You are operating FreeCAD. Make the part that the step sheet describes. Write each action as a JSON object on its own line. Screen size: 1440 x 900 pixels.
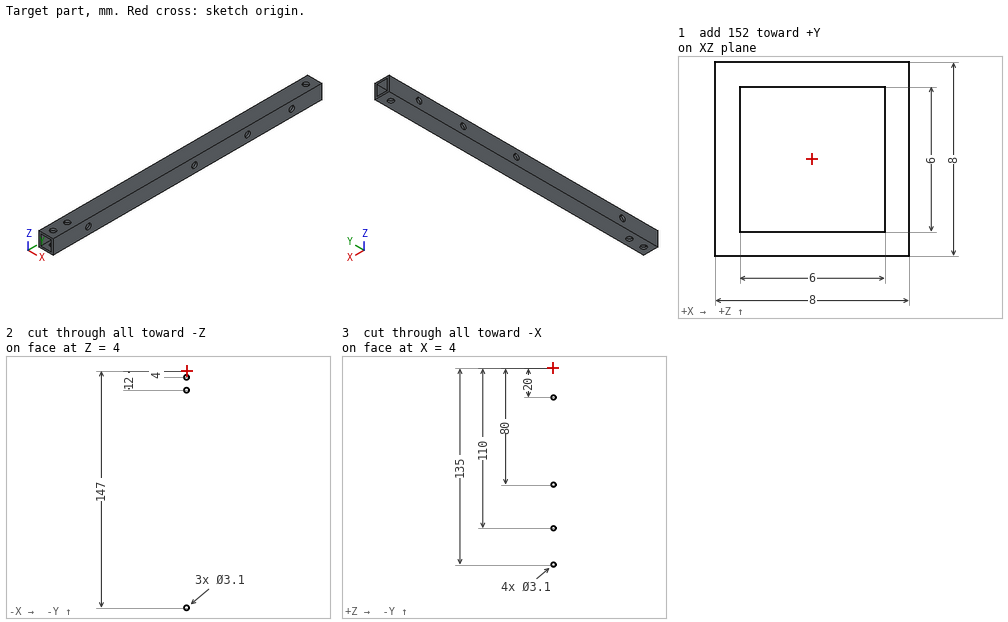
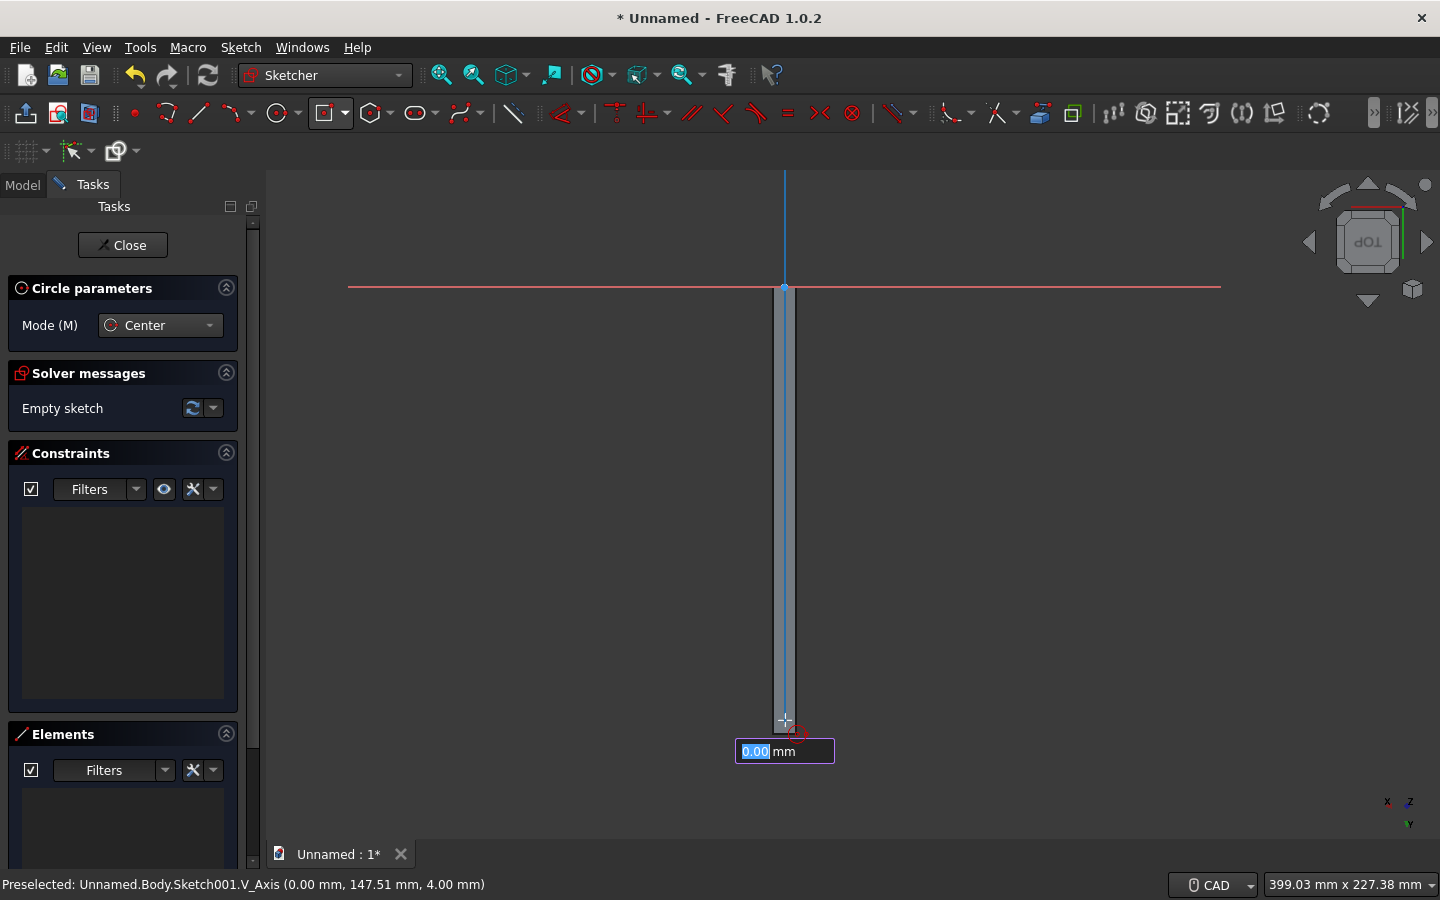
{"action": "scroll", "coordinate": [789, 718], "scroll_direction": "up", "scroll_amount": 7}
{"action": "mouse_move", "coordinate": [787, 715]}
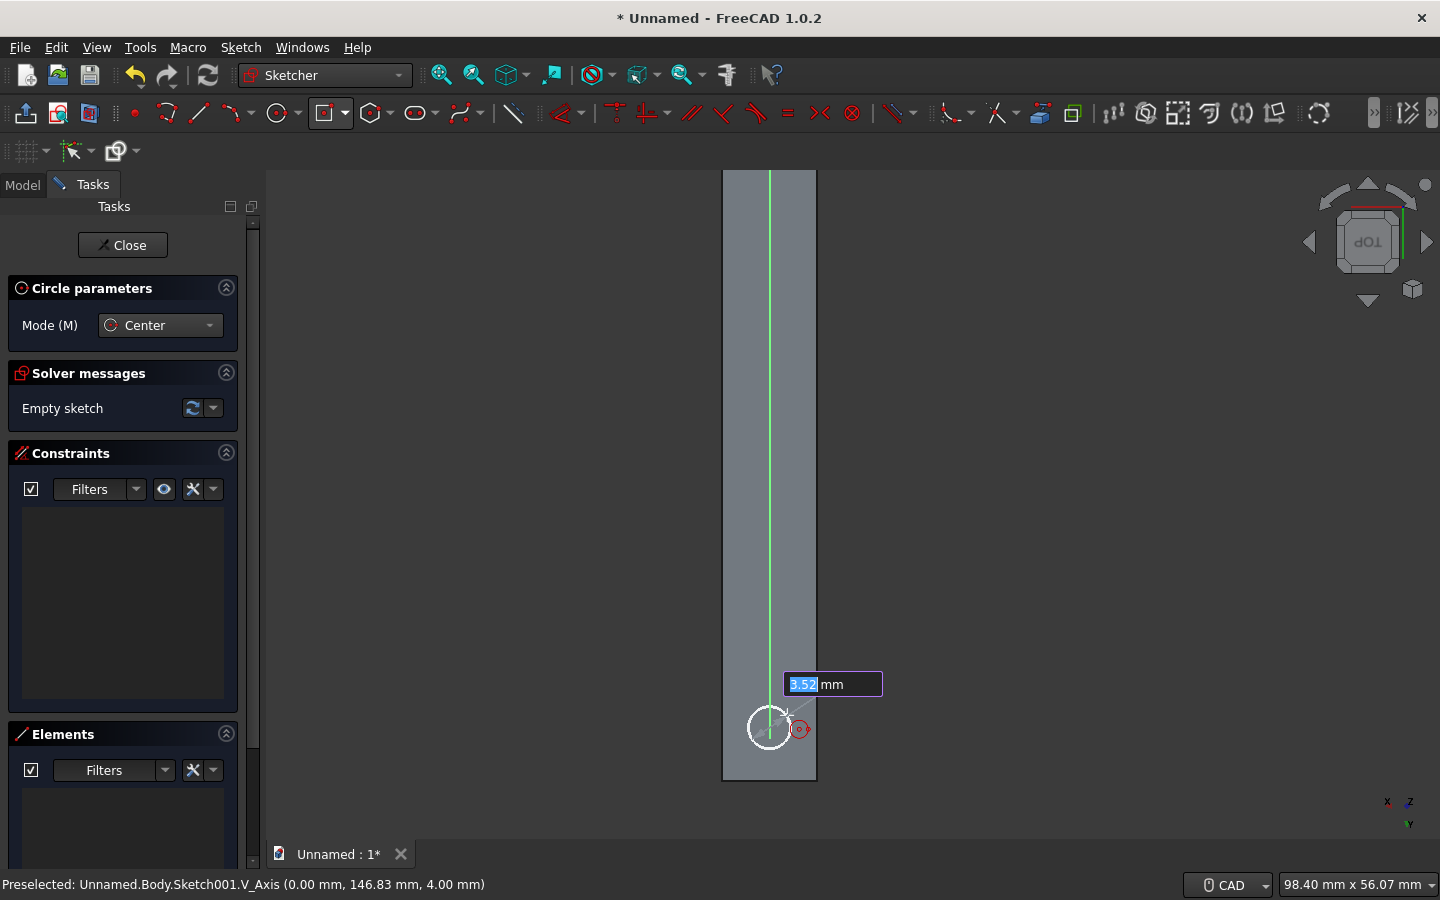
{"action": "type", "text": "3.1"}
{"action": "key", "text": "Return"}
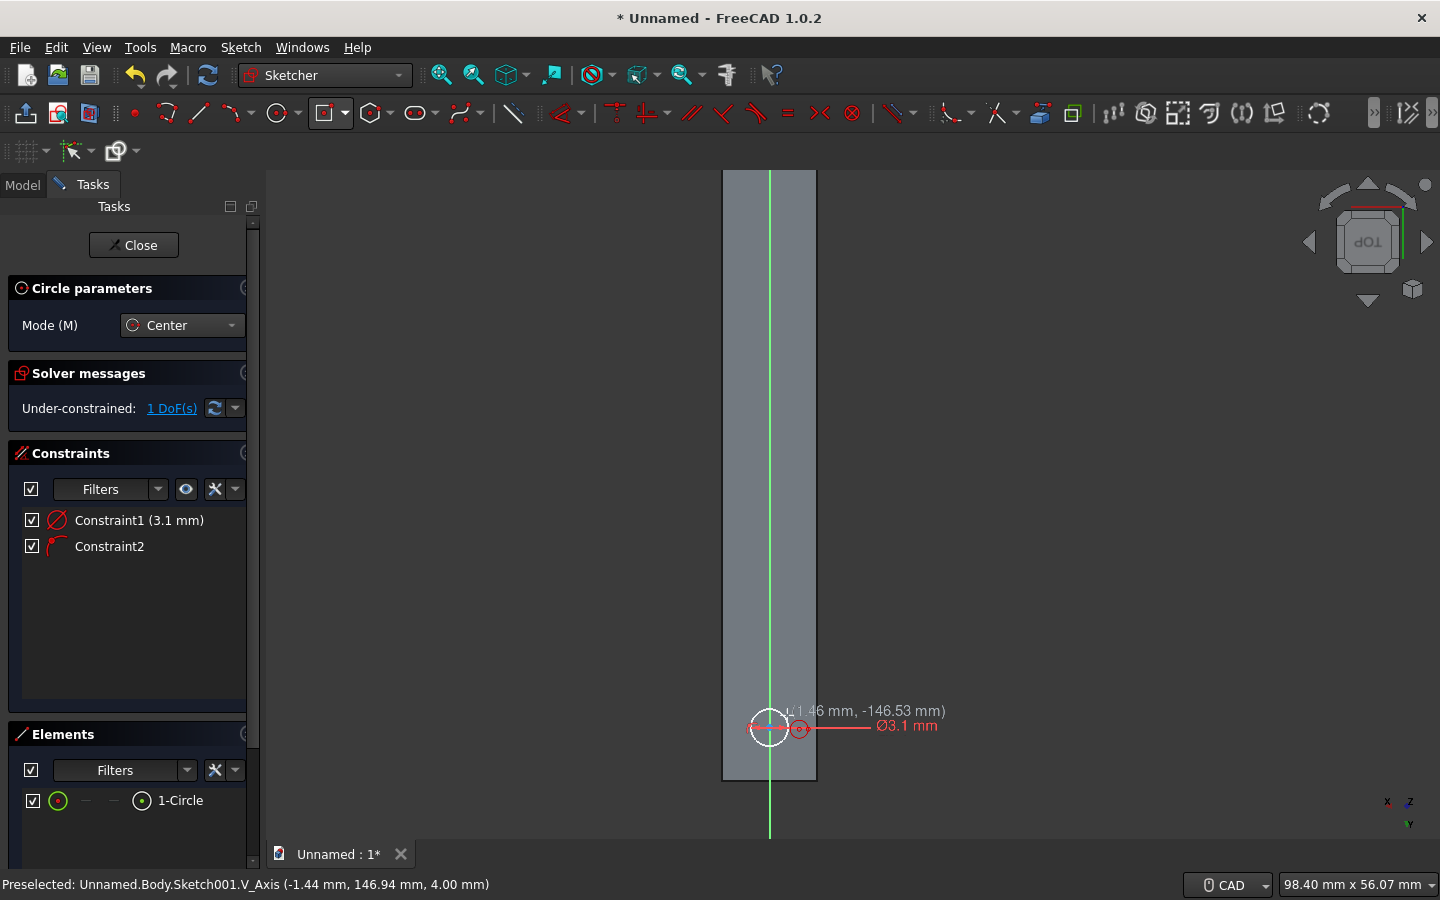
{"action": "scroll", "coordinate": [789, 717], "scroll_direction": "down", "scroll_amount": 7}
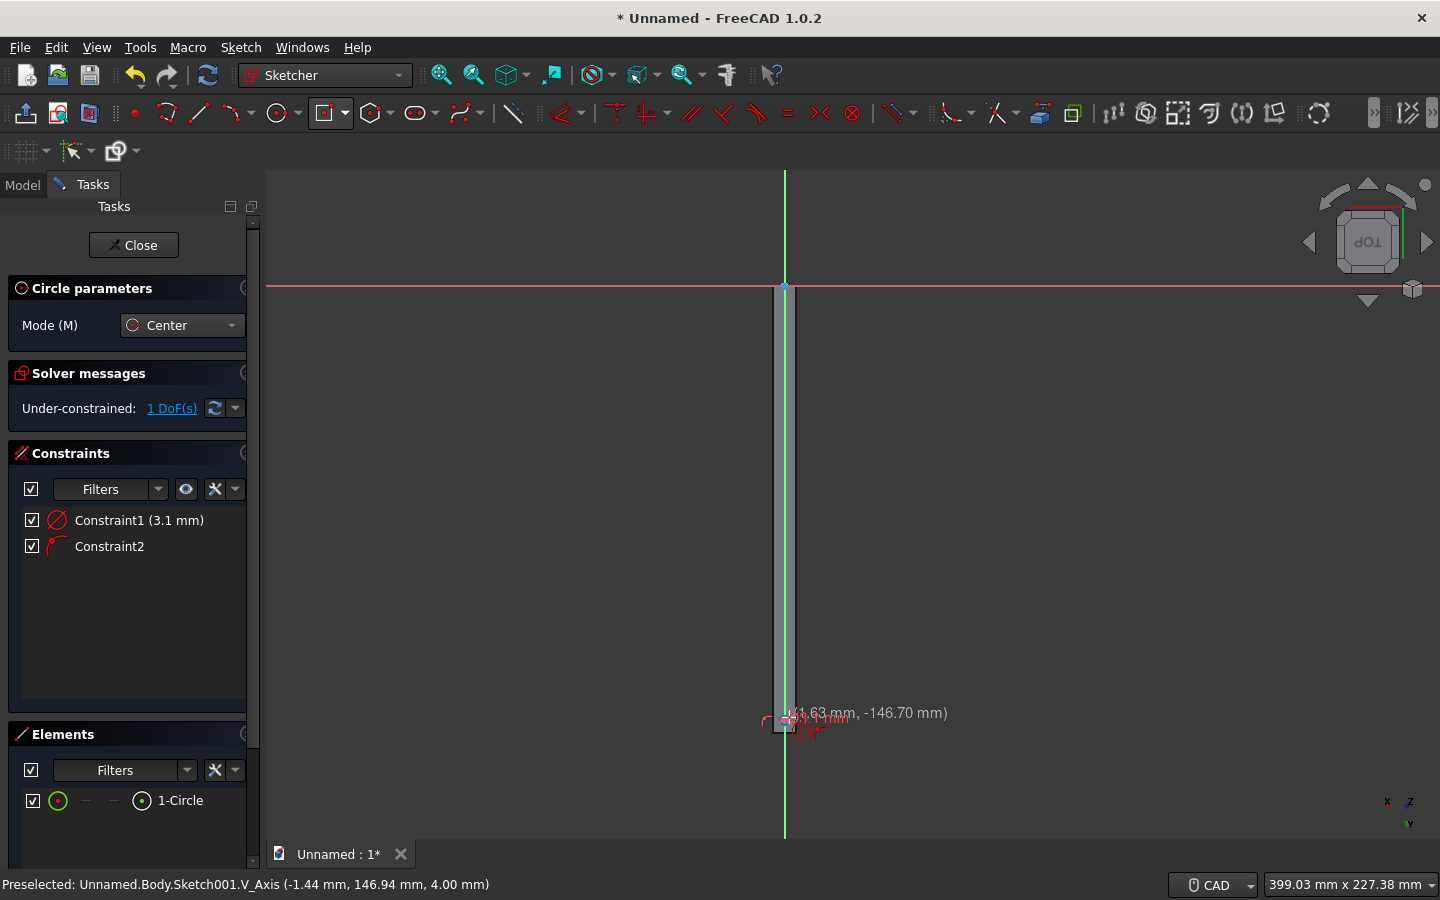
{"action": "scroll", "coordinate": [785, 298], "scroll_direction": "up", "scroll_amount": 9}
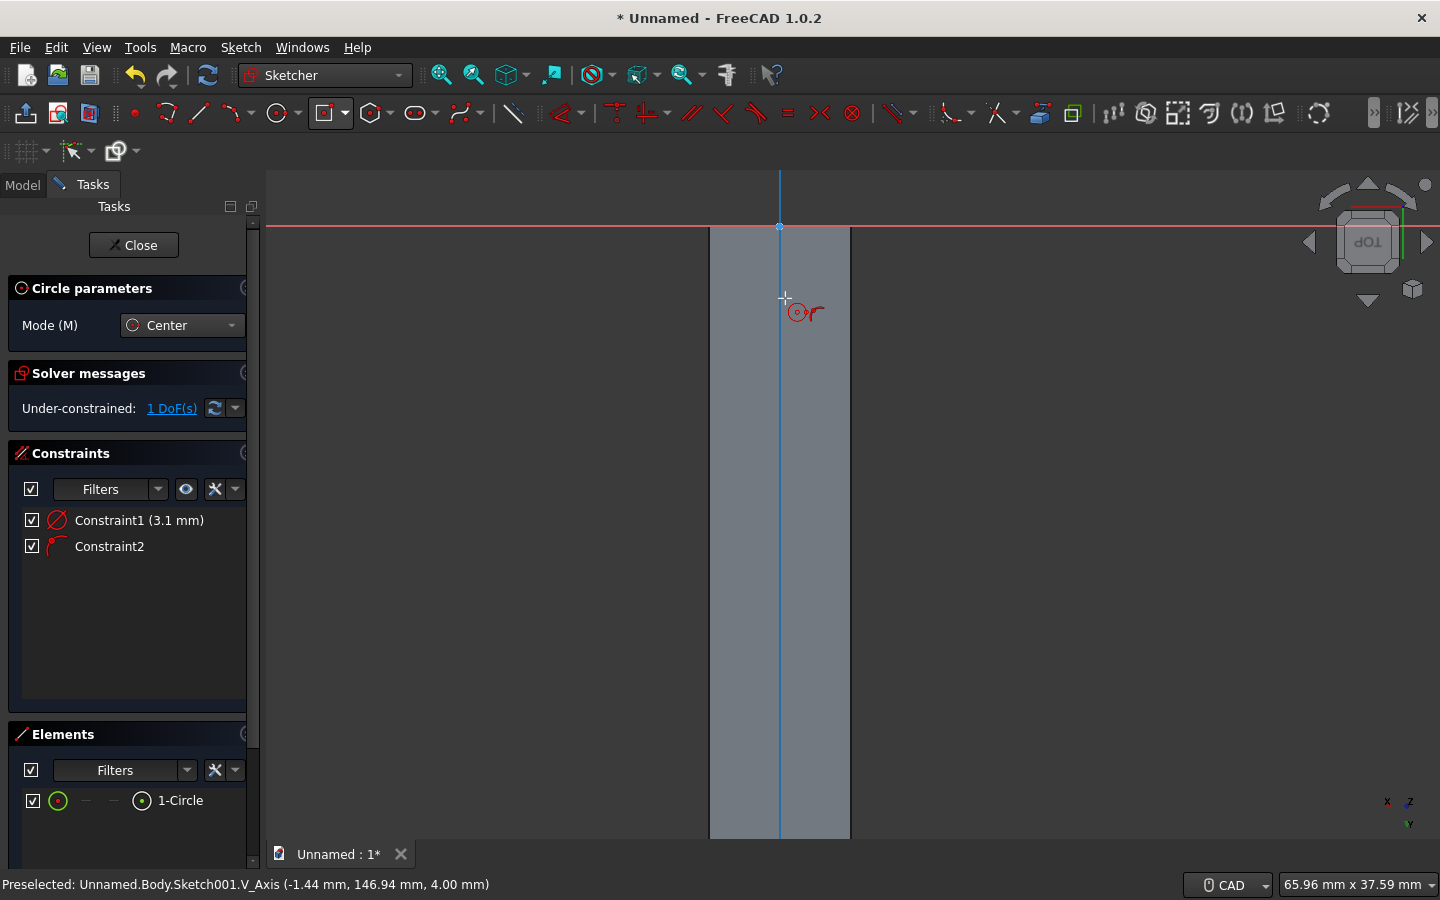
{"action": "scroll", "coordinate": [785, 298], "scroll_direction": "down", "scroll_amount": 9}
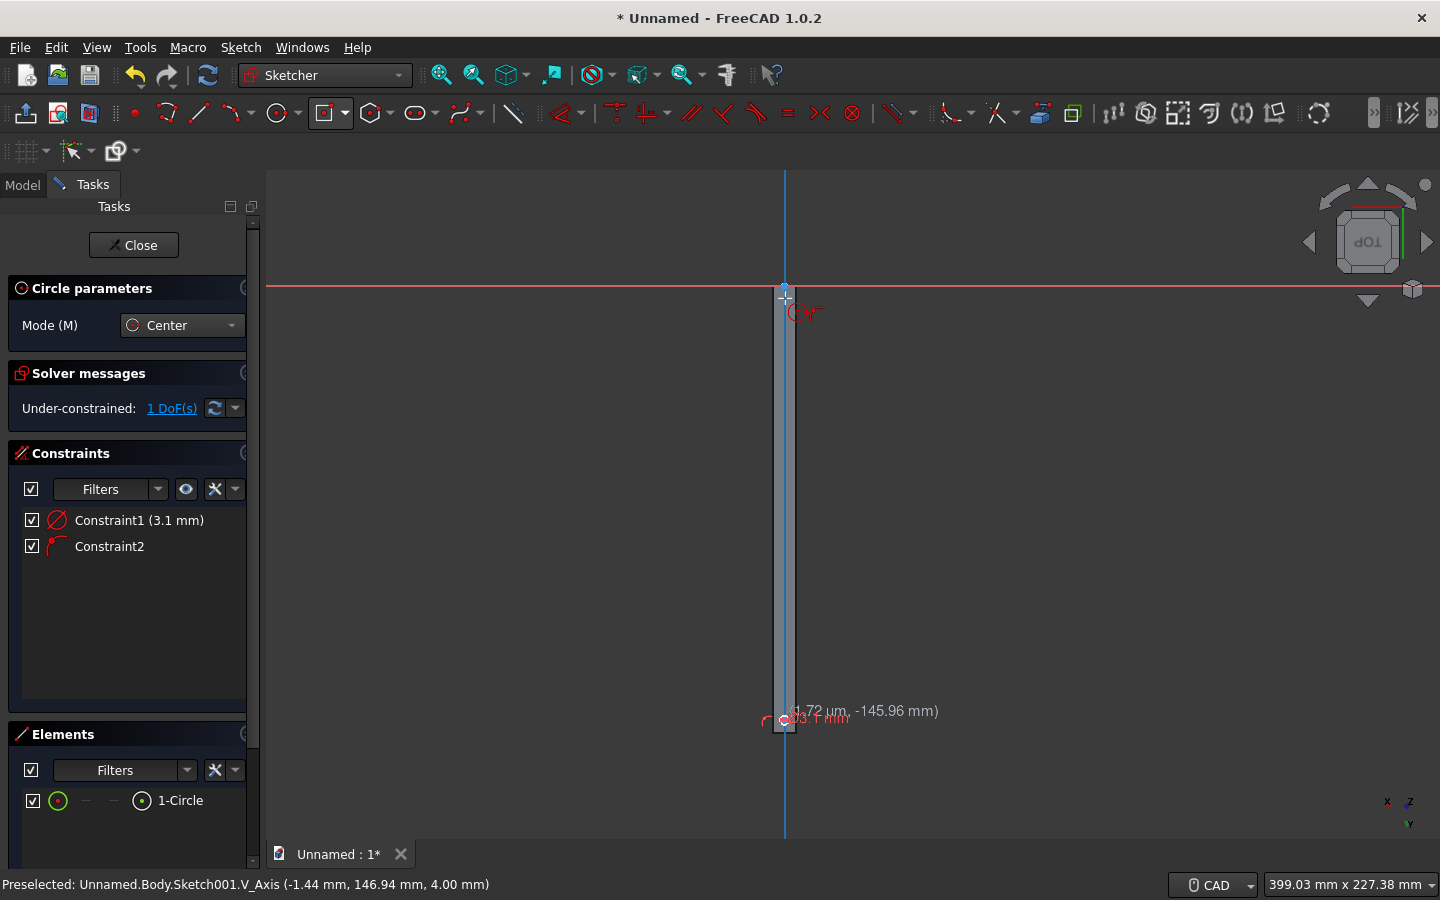
{"action": "scroll", "coordinate": [785, 298], "scroll_direction": "up", "scroll_amount": 2}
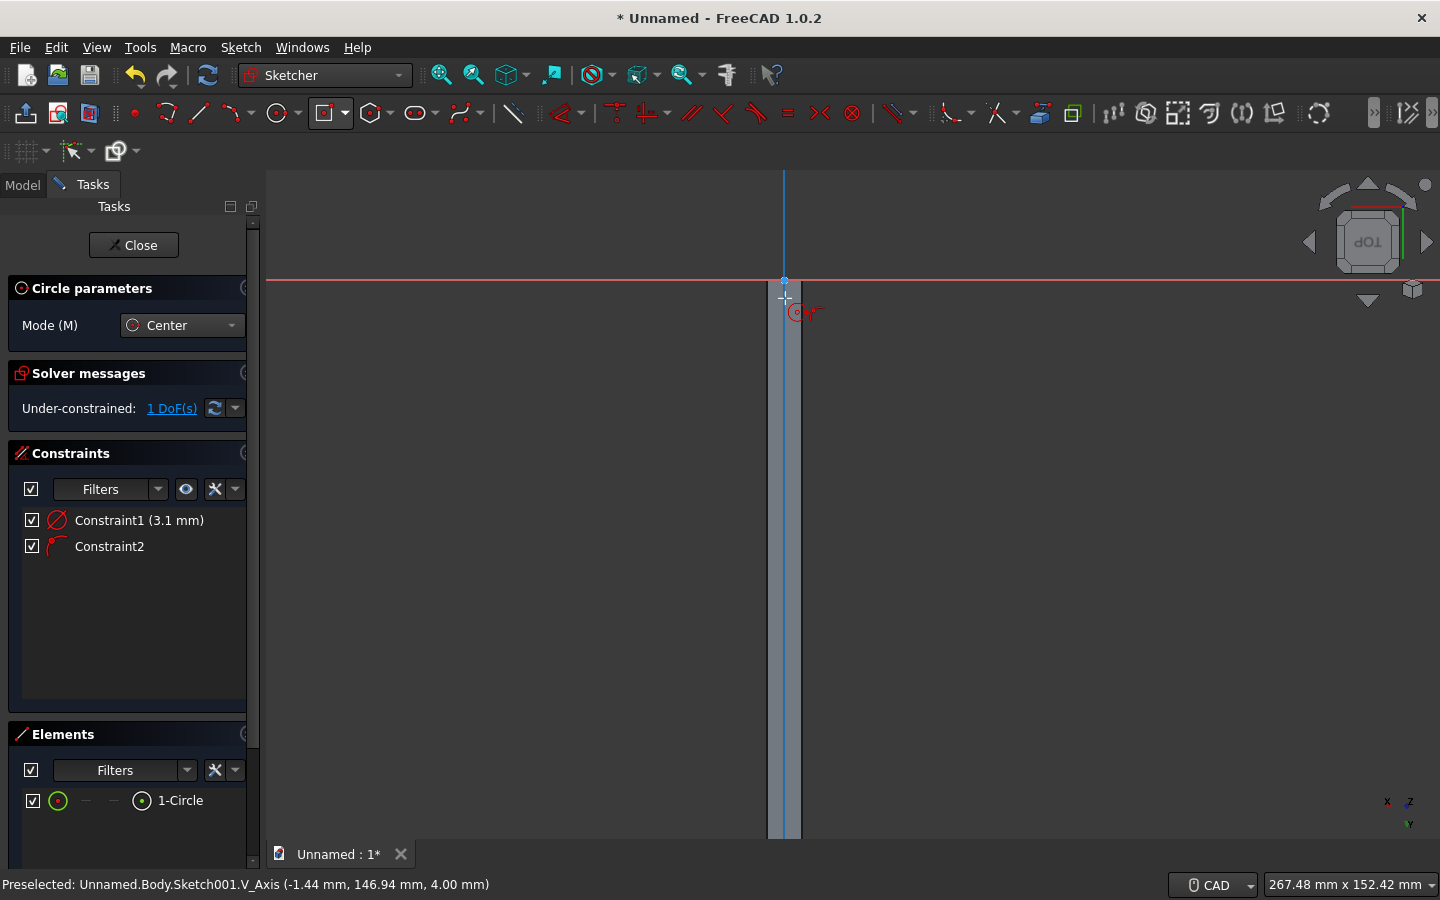
{"action": "left_click", "coordinate": [784, 298]}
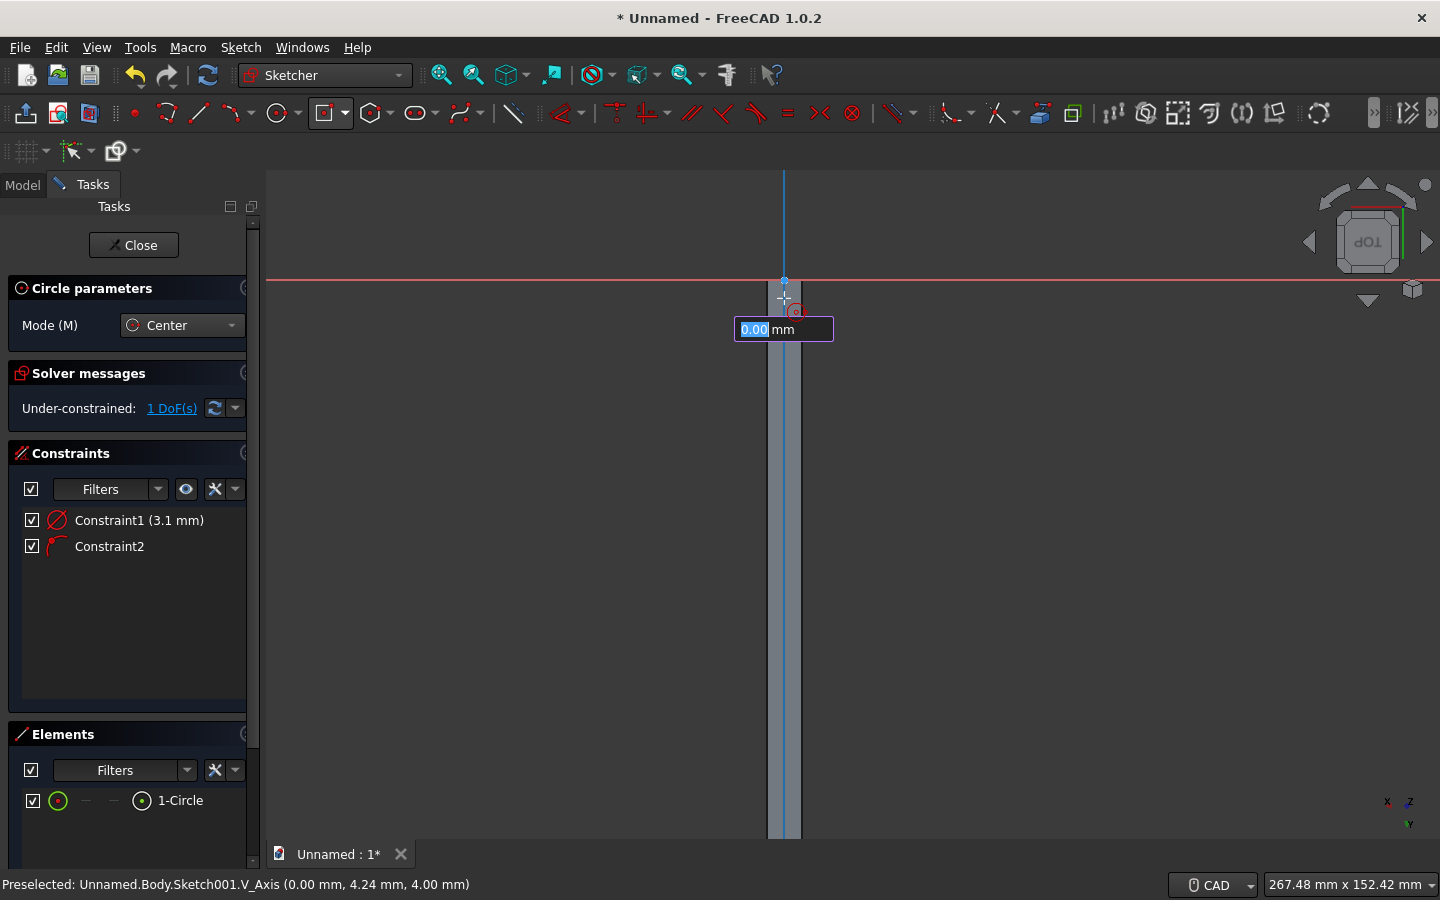
{"action": "scroll", "coordinate": [790, 296], "scroll_direction": "up", "scroll_amount": 5}
{"action": "mouse_move", "coordinate": [791, 295]}